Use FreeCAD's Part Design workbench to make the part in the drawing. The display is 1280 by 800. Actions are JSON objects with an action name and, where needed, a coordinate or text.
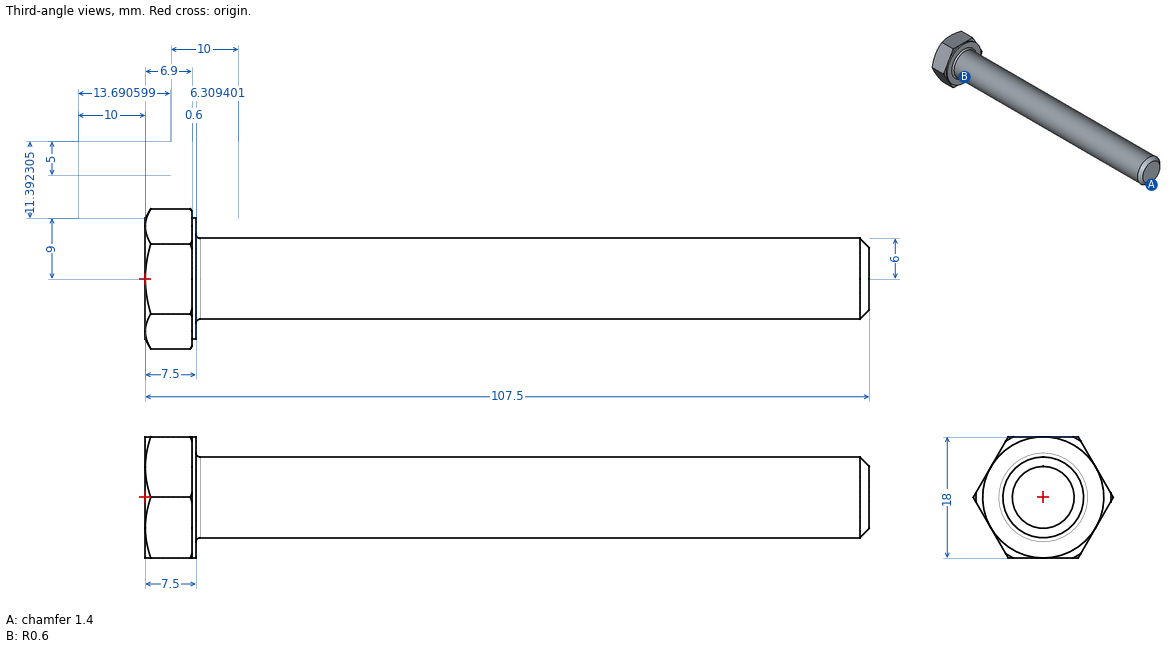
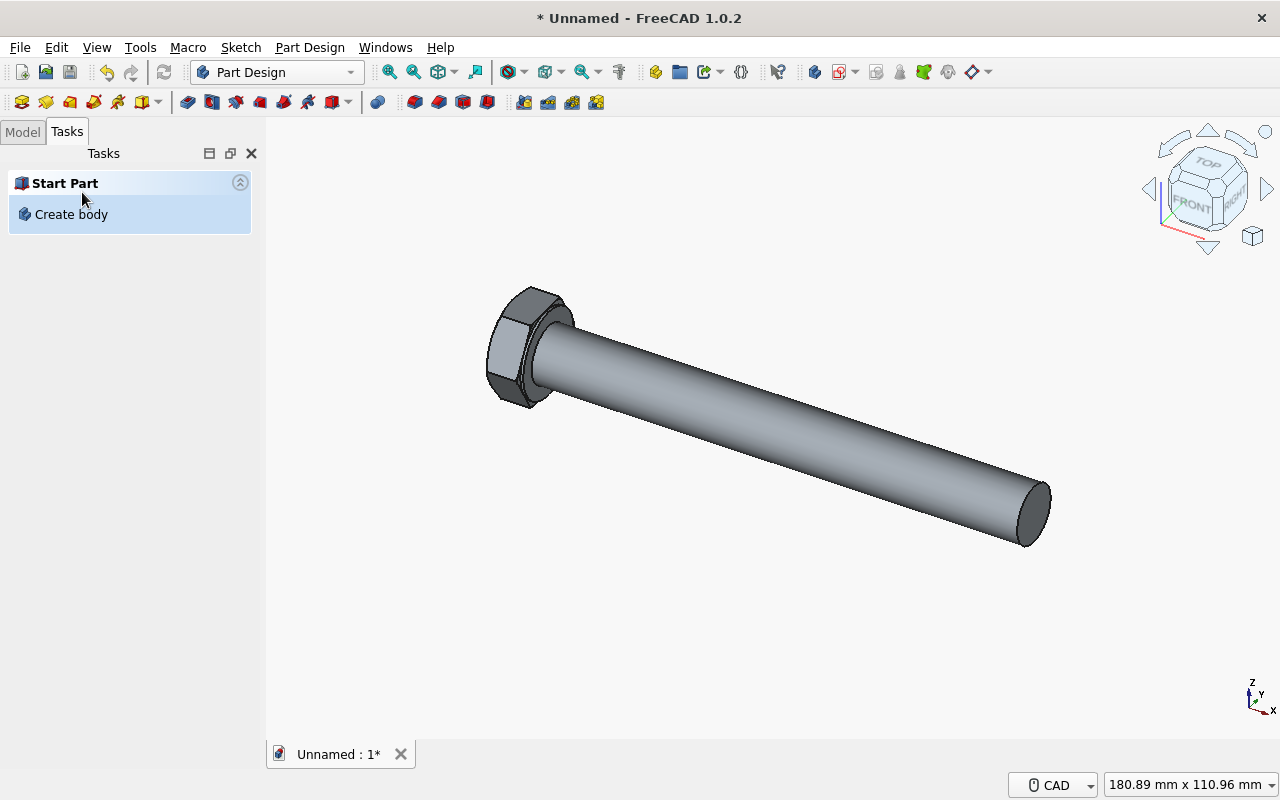
{"action": "left_click", "coordinate": [1017, 530]}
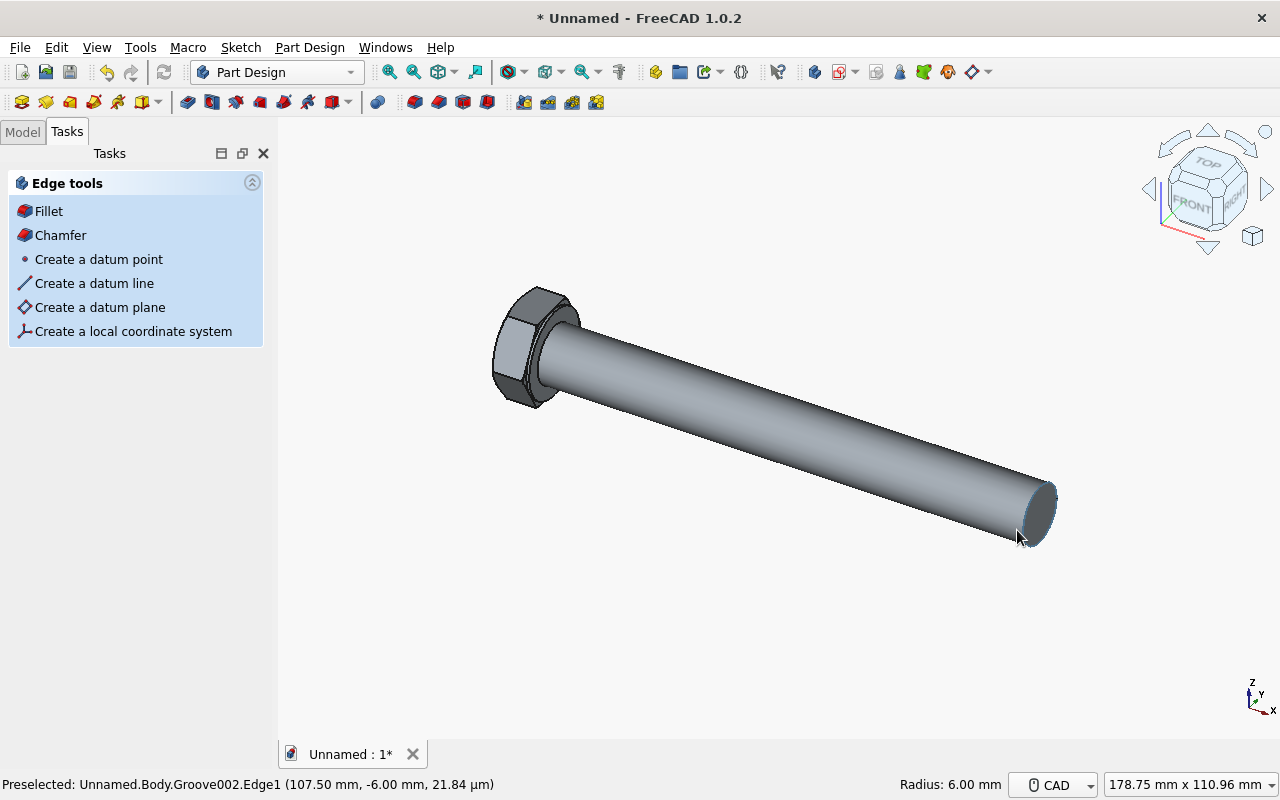
{"action": "left_click", "coordinate": [440, 102]}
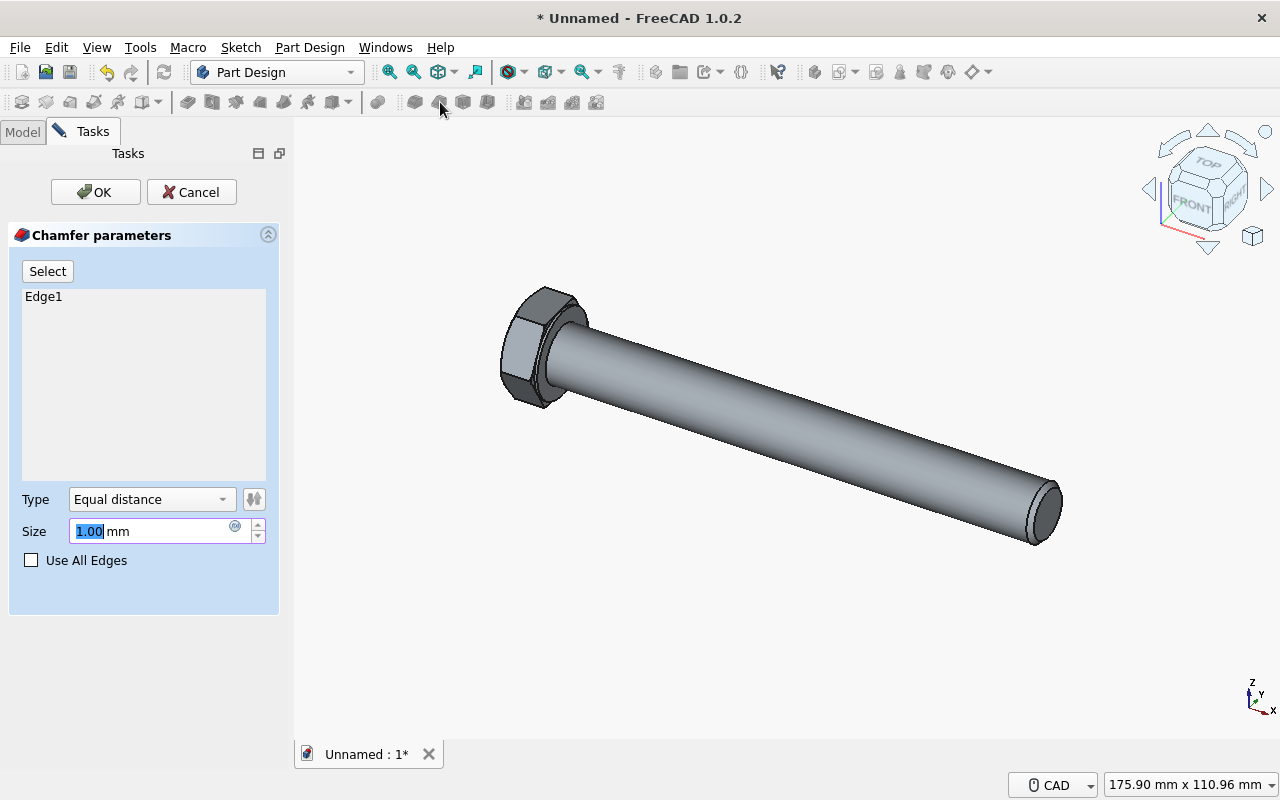
{"action": "type", "text": "1.4"}
{"action": "key", "text": "Tab"}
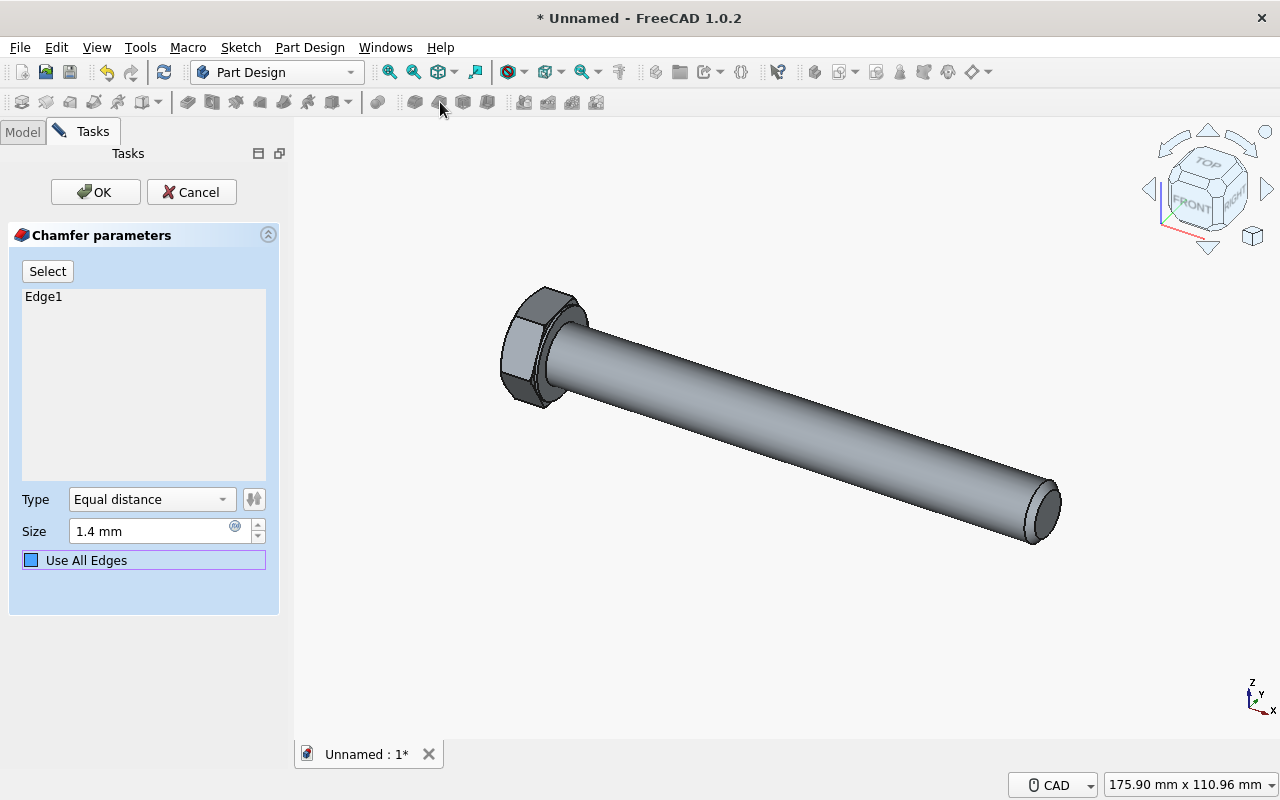
{"action": "left_click", "coordinate": [96, 192]}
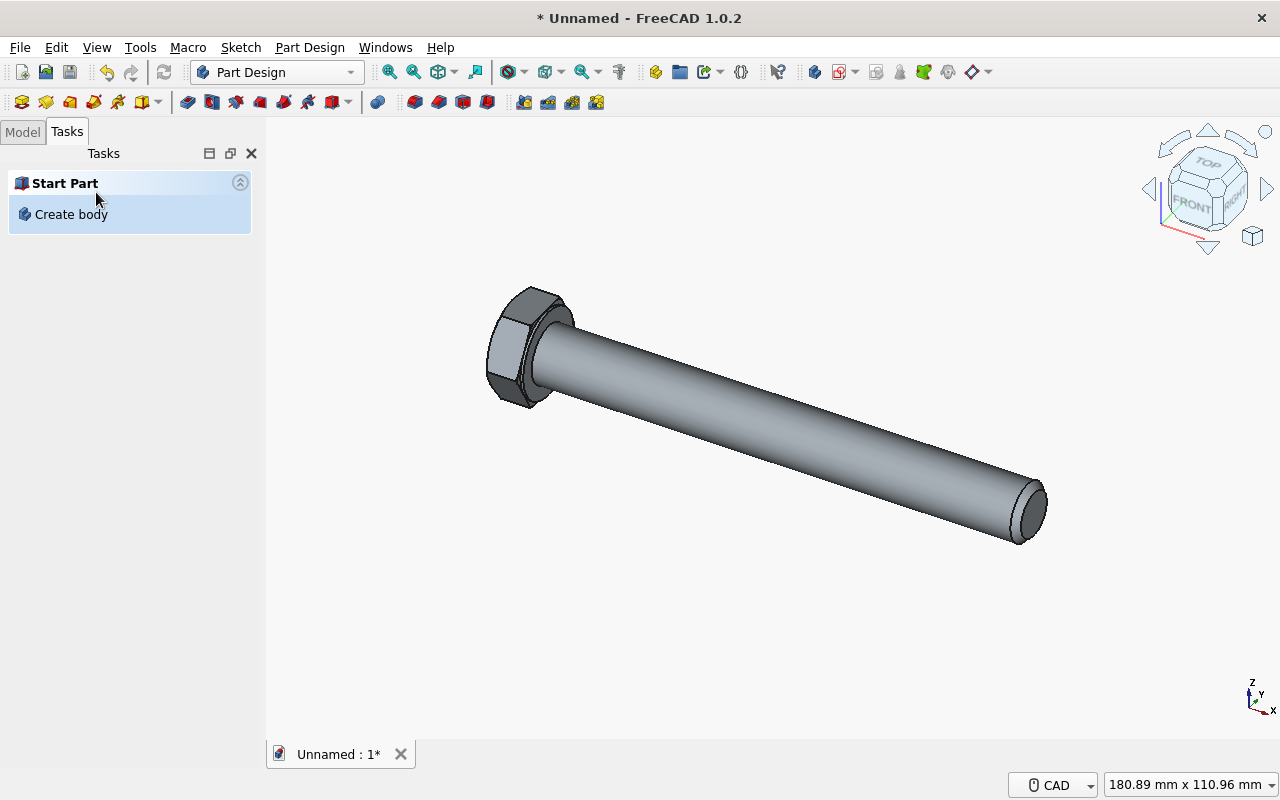
{"action": "key", "text": "0"}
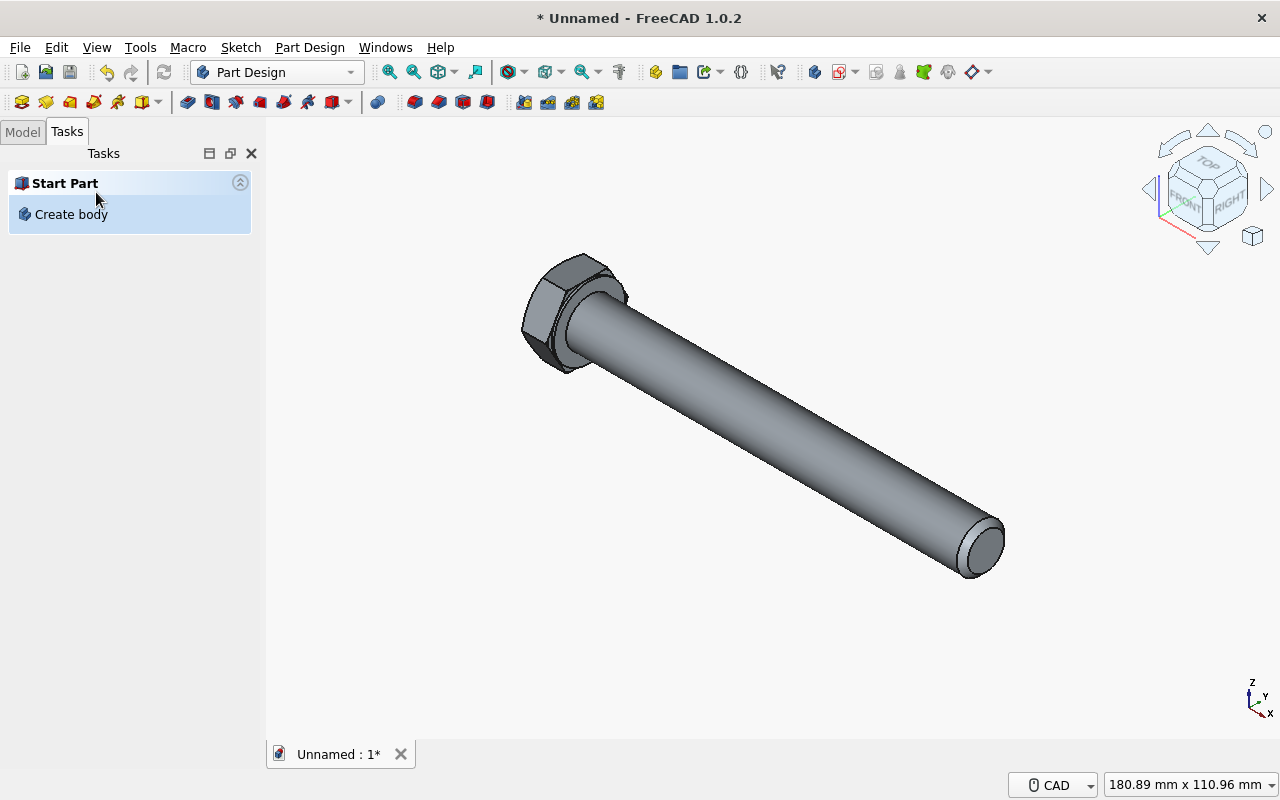
{"action": "key", "text": "2"}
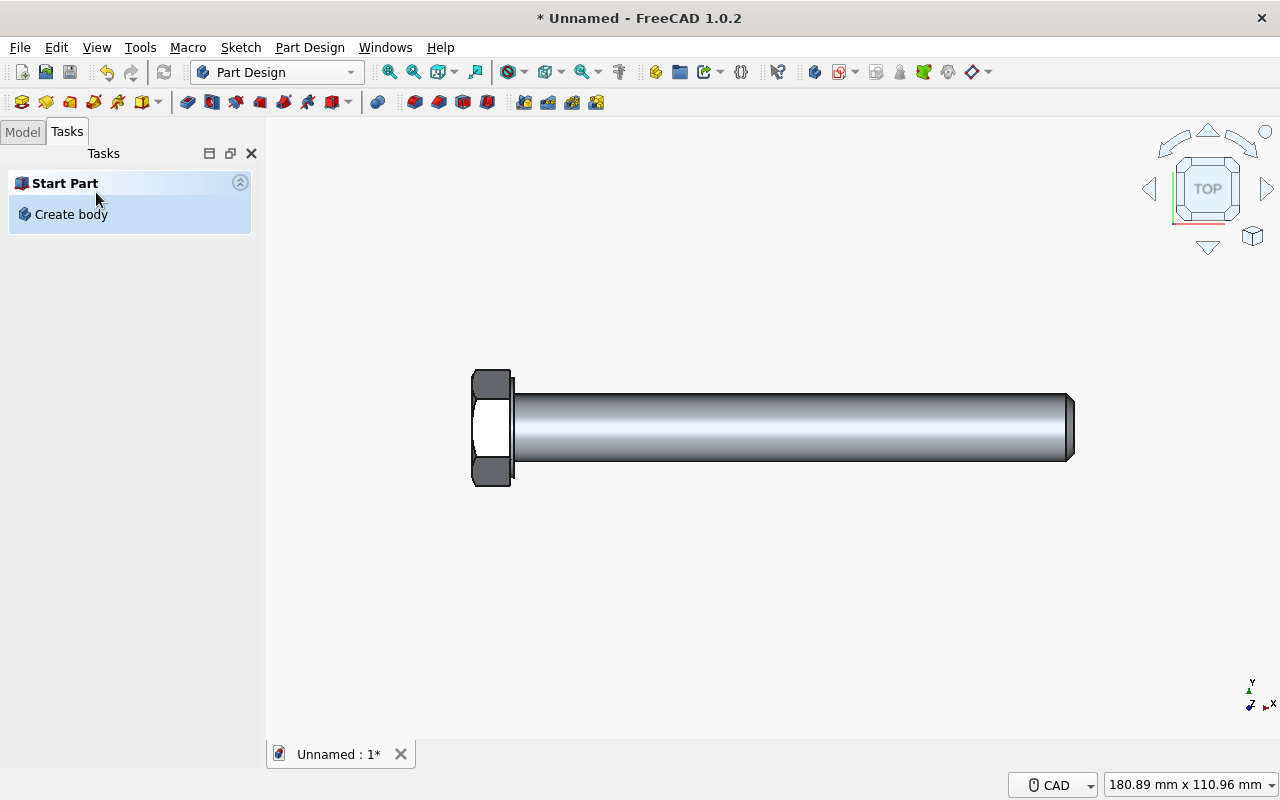
{"action": "key", "text": "1"}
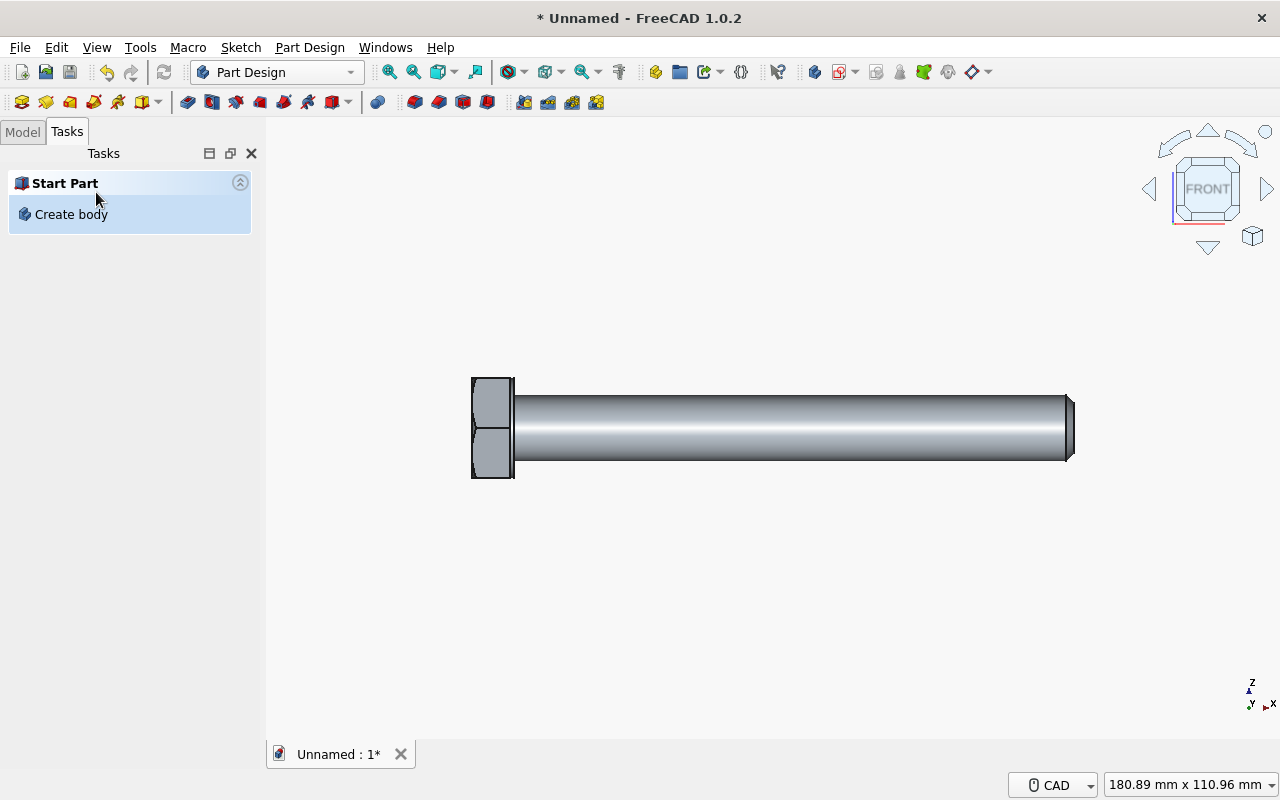
{"action": "key", "text": "3"}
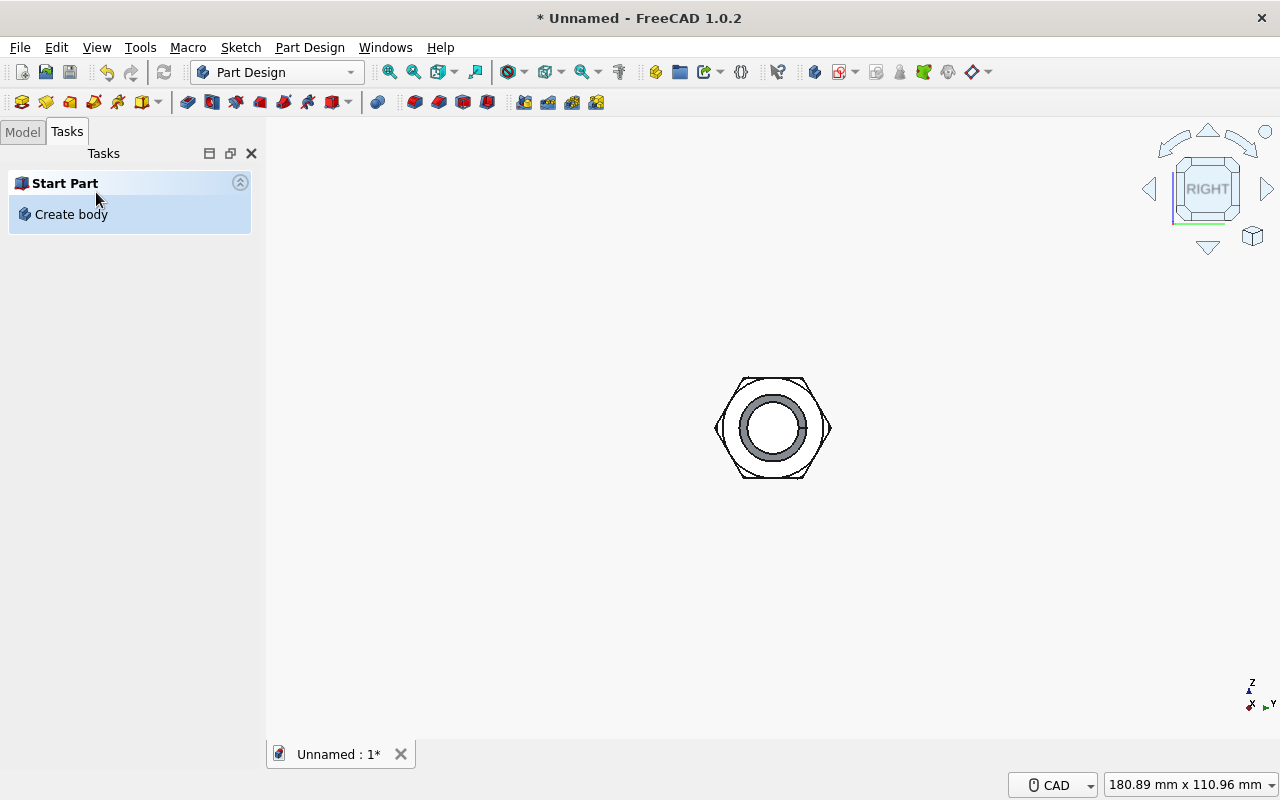
{"action": "key", "text": "v f"}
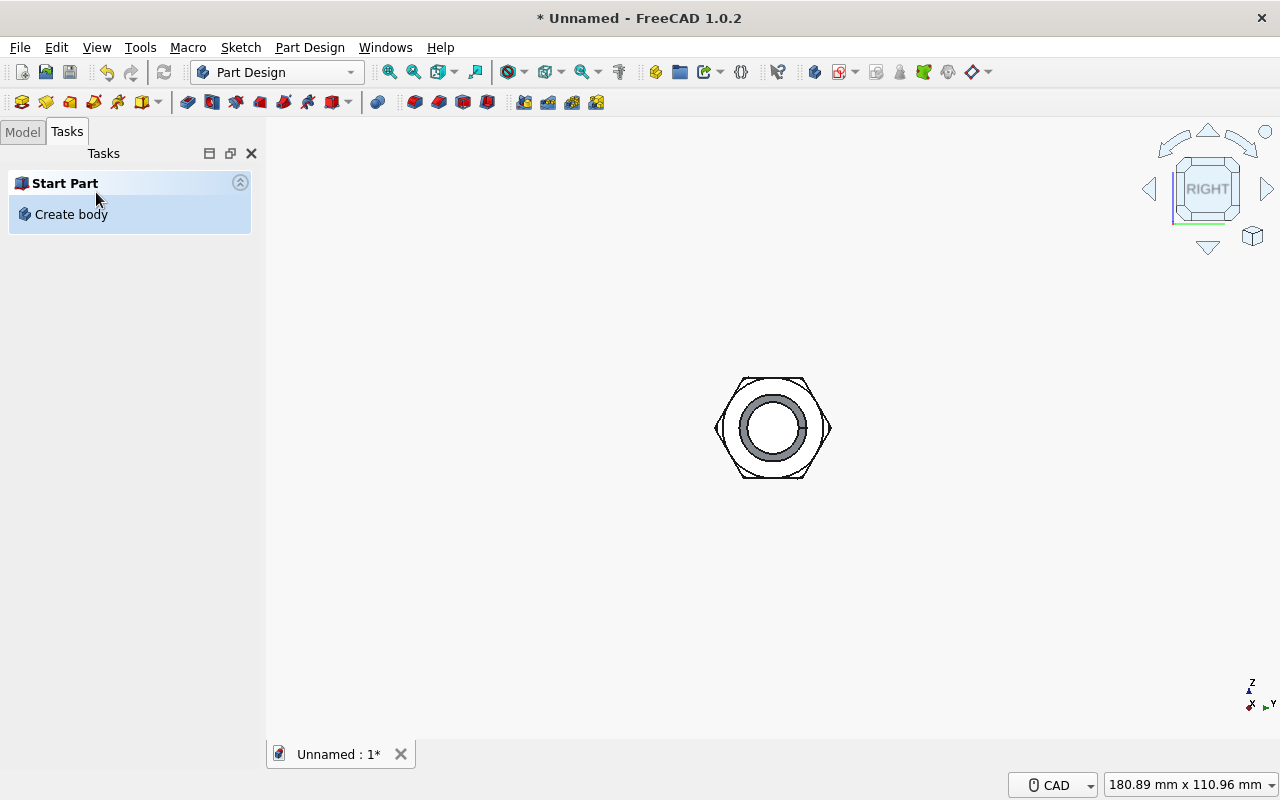
{"action": "key", "text": "5"}